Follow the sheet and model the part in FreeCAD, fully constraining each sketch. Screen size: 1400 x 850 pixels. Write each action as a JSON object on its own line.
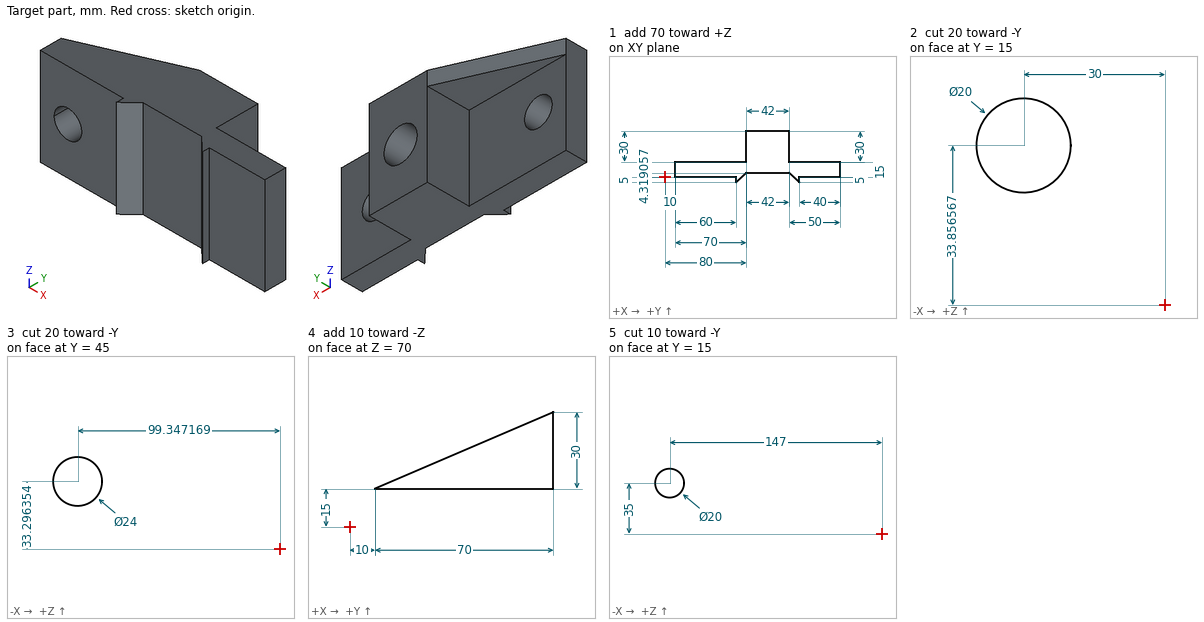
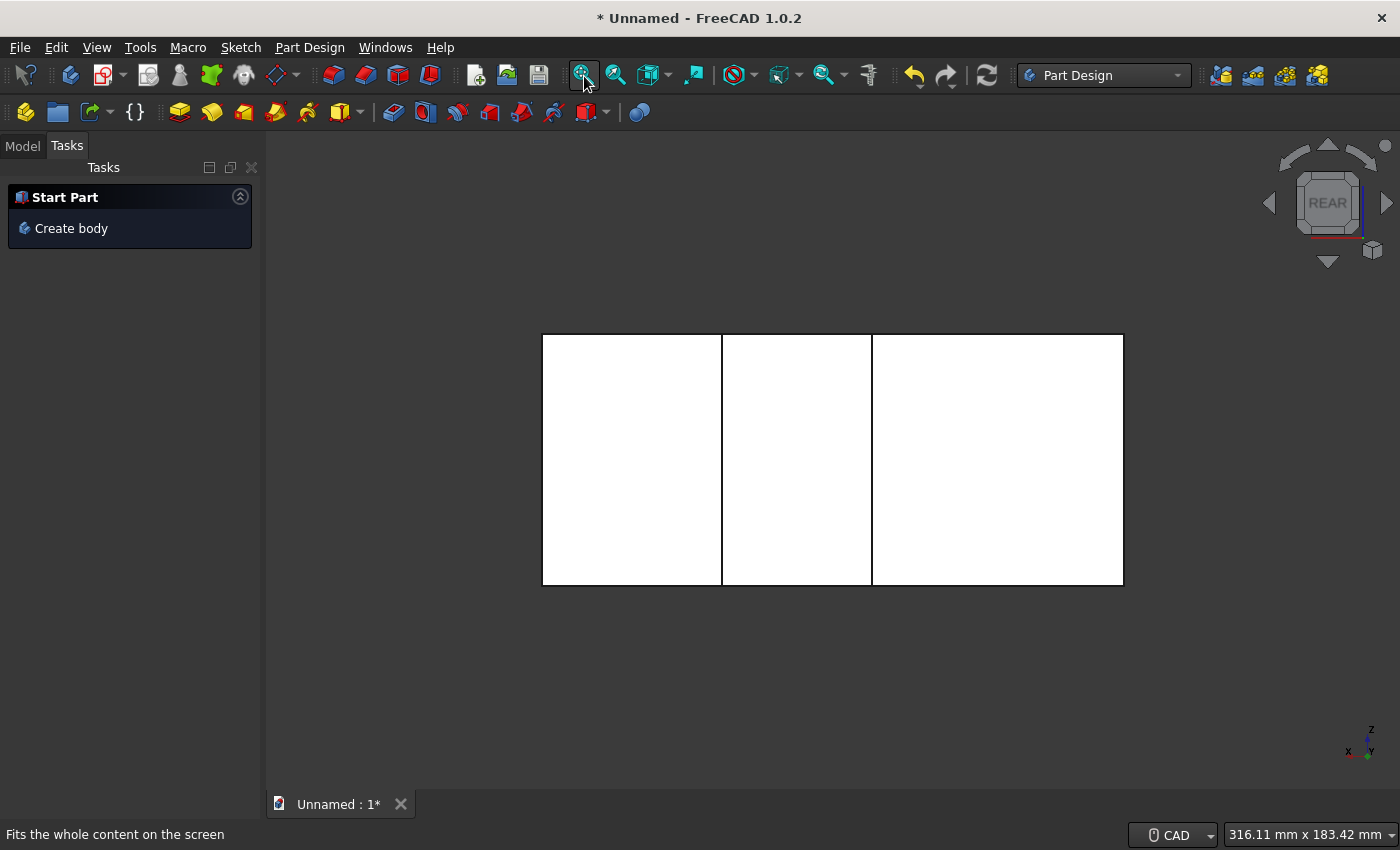
{"action": "left_click", "coordinate": [998, 459]}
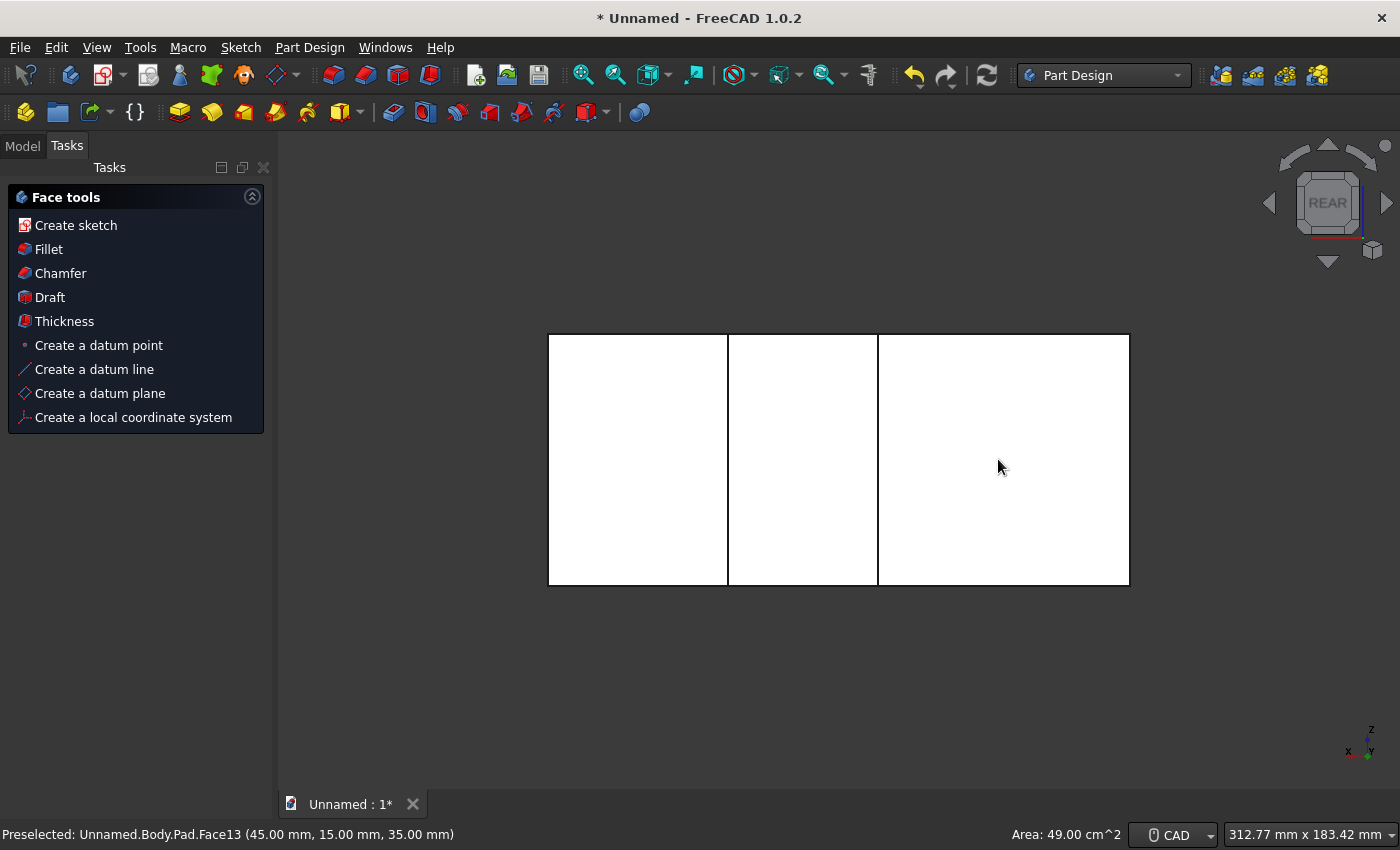
{"action": "left_click", "coordinate": [104, 76]}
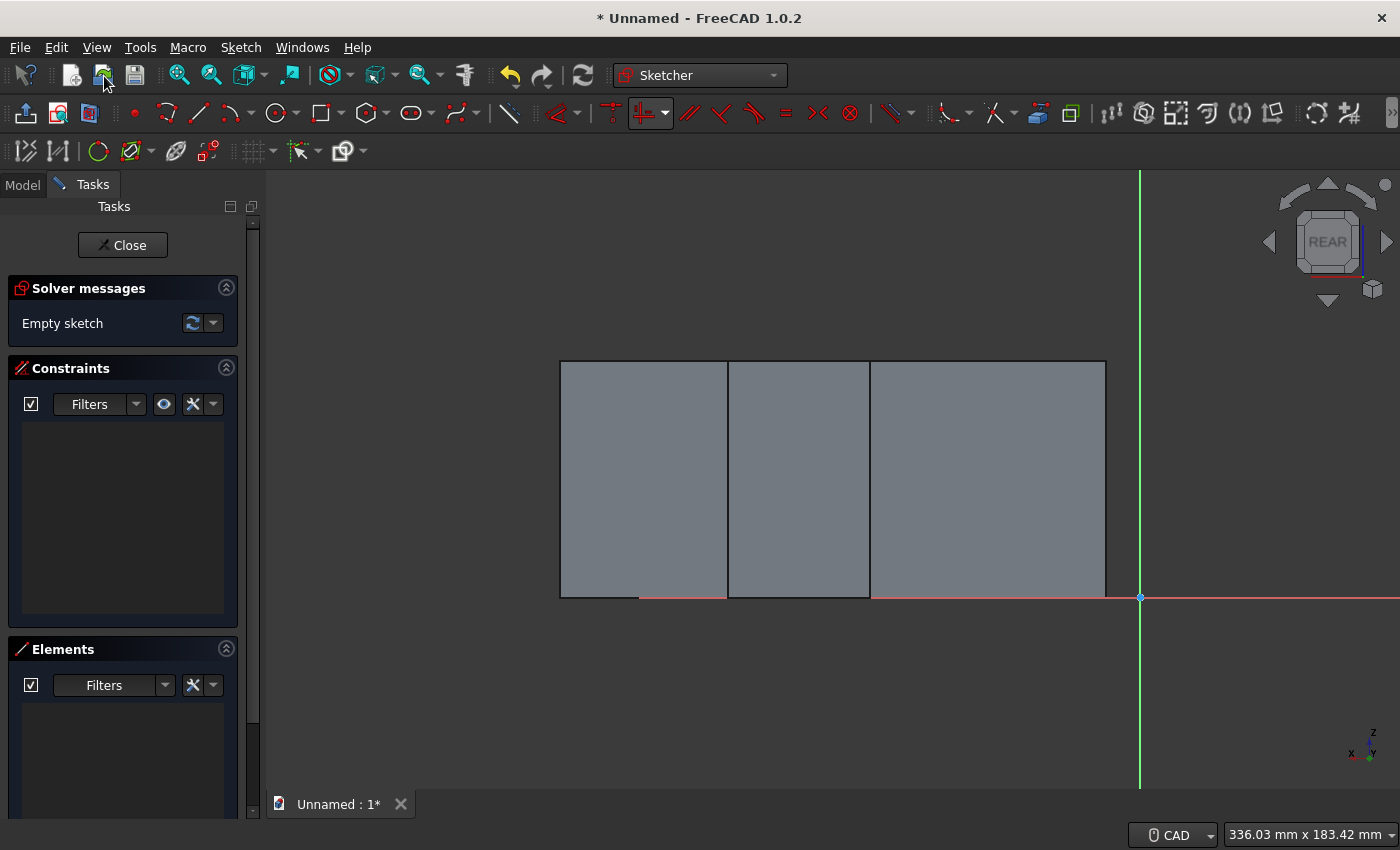
{"action": "left_click", "coordinate": [90, 114]}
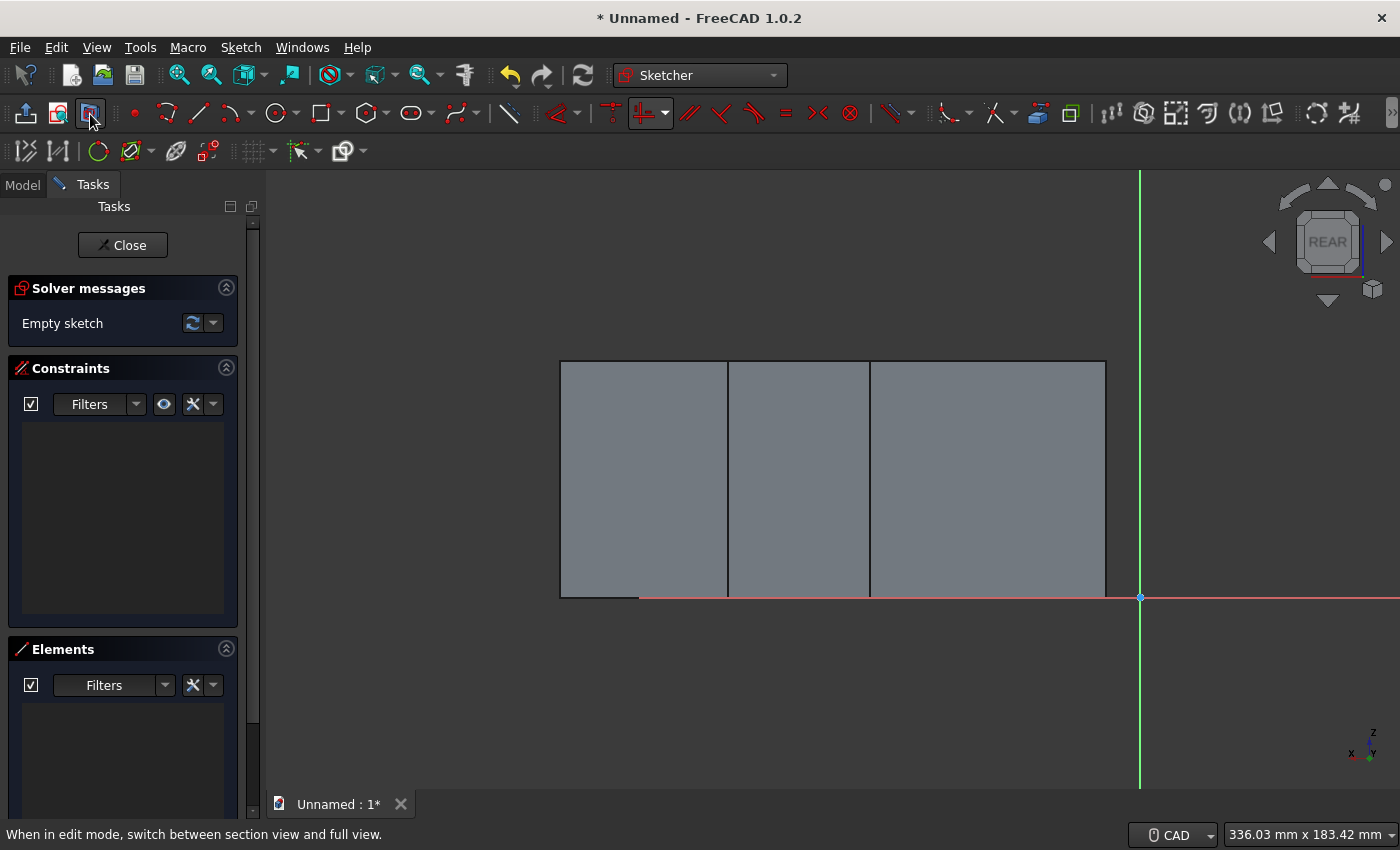
{"action": "scroll", "coordinate": [1235, 549], "scroll_direction": "up", "scroll_amount": 5}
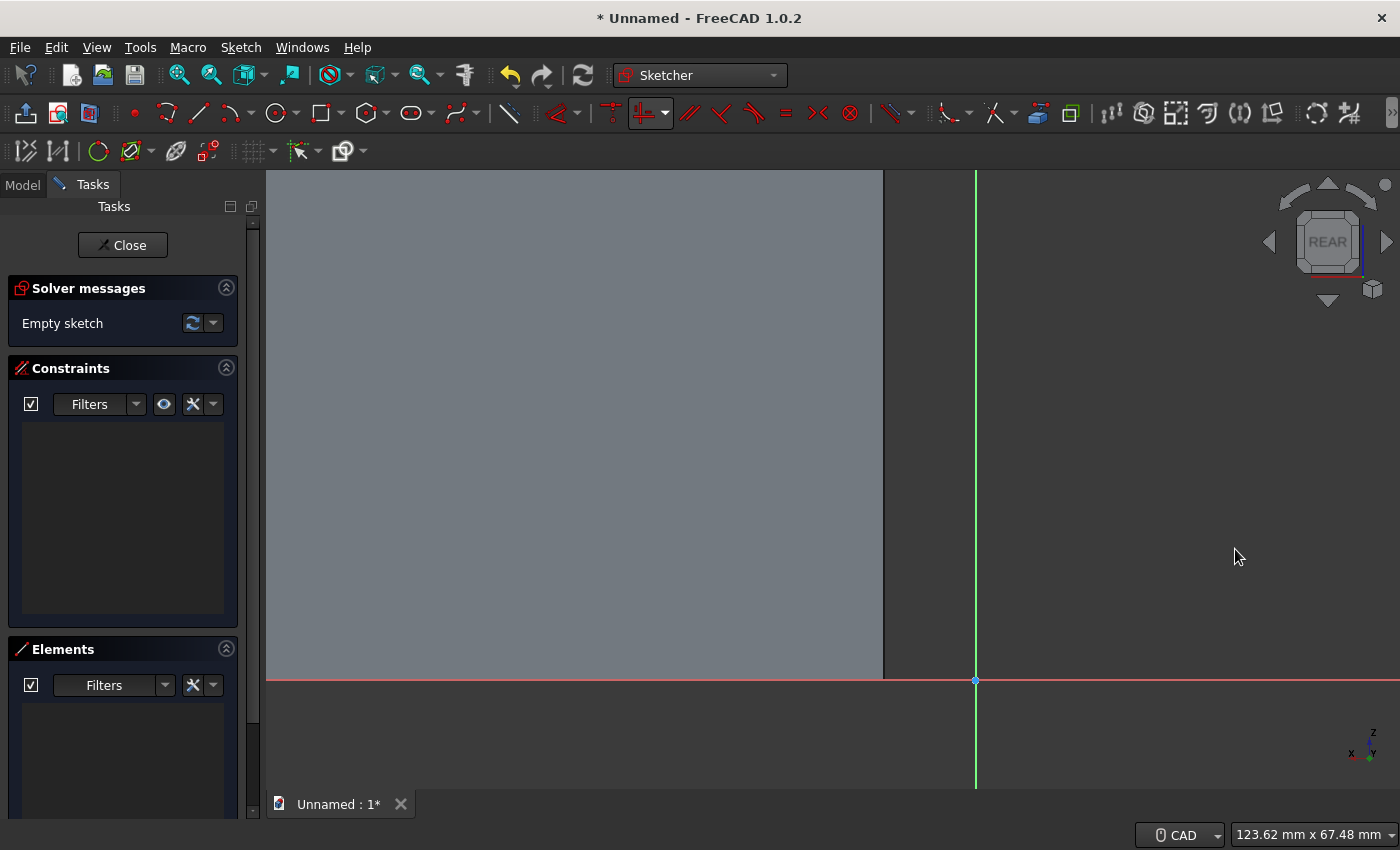
{"action": "left_click", "coordinate": [276, 114]}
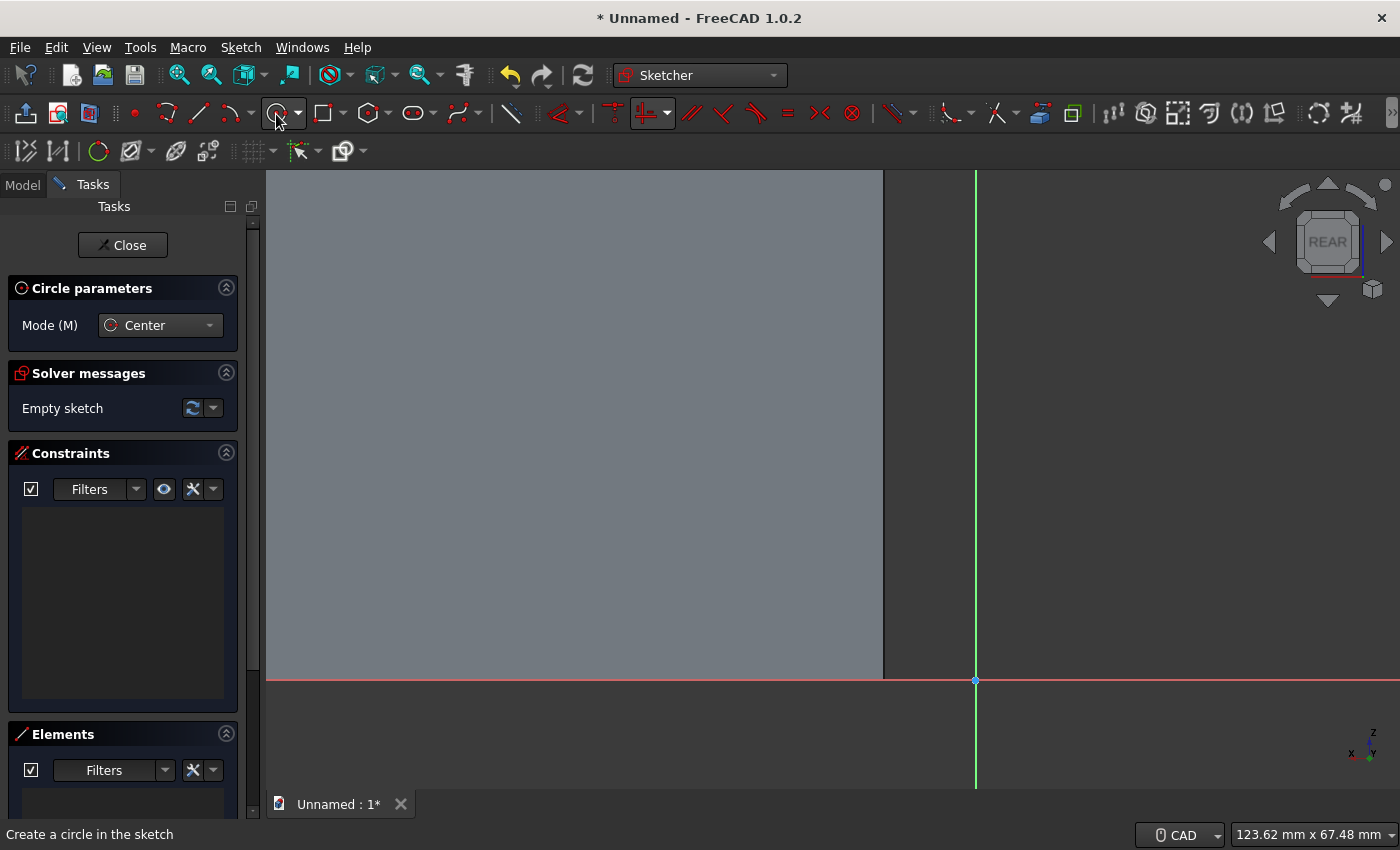
{"action": "left_click", "coordinate": [700, 370]}
{"action": "mouse_move", "coordinate": [765, 305]}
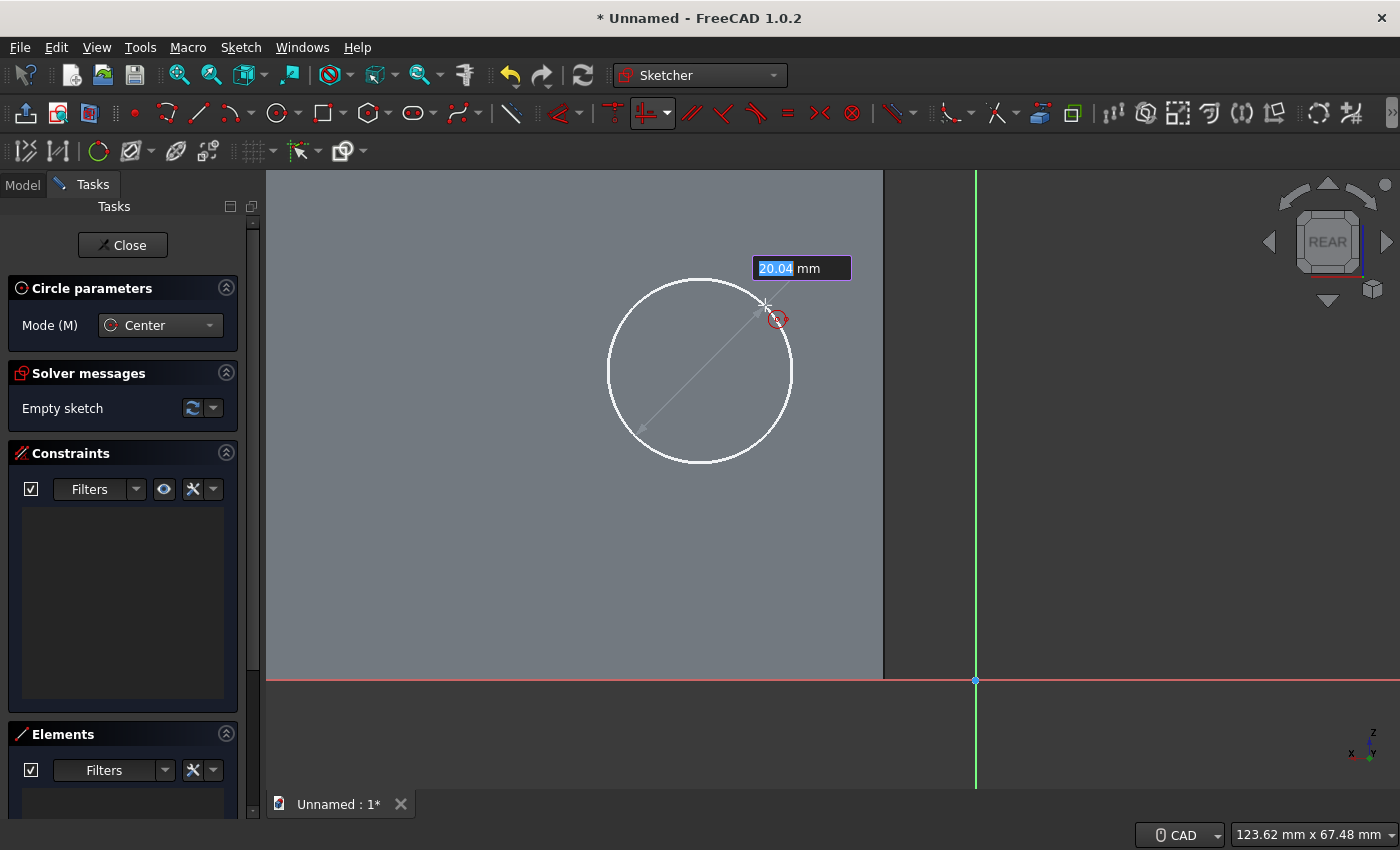
{"action": "type", "text": "20"}
{"action": "key", "text": "Return"}
{"action": "key", "text": "Escape"}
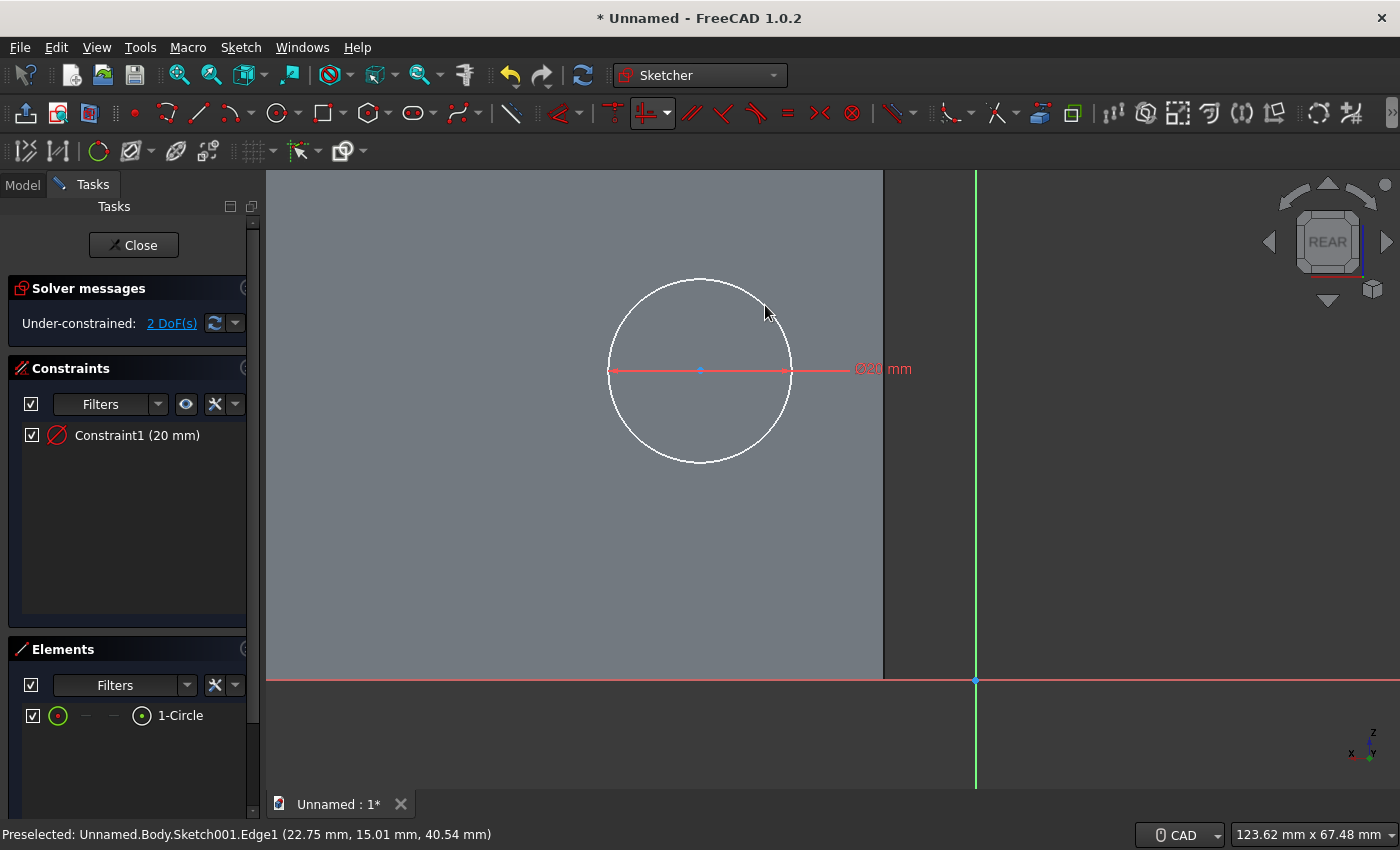
{"action": "left_click", "coordinate": [558, 114]}